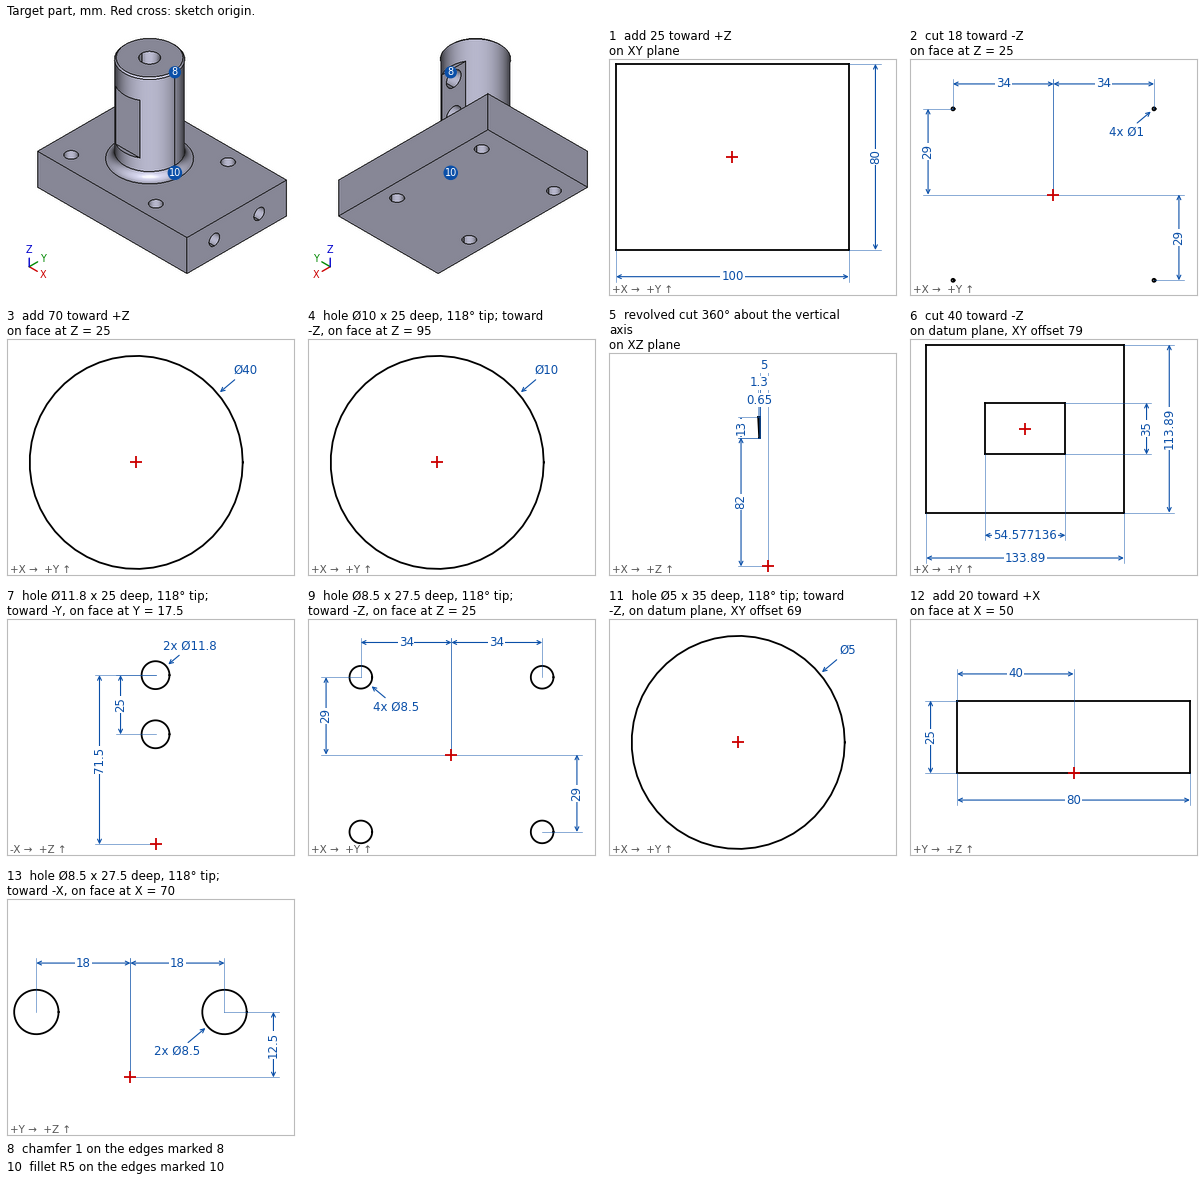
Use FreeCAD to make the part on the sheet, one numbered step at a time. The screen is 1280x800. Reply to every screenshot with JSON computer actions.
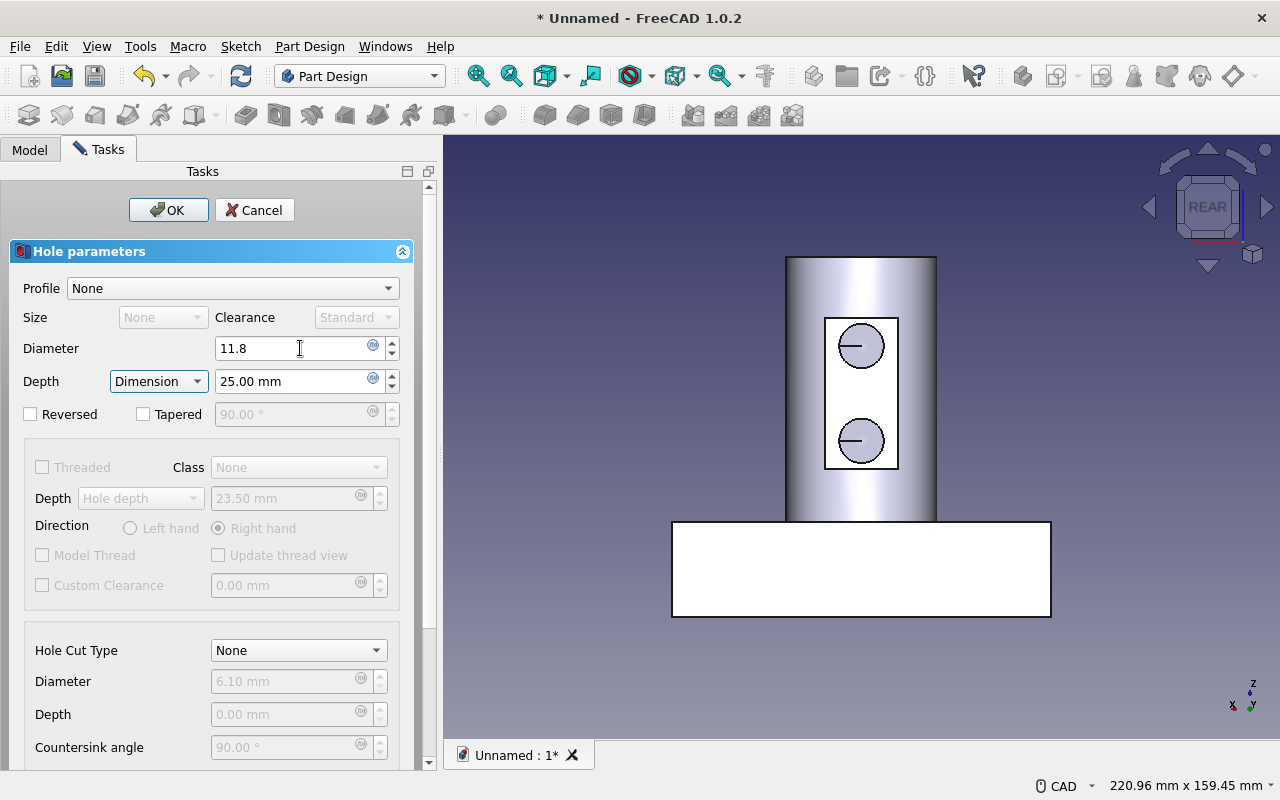
{"action": "triple_click", "coordinate": [300, 382]}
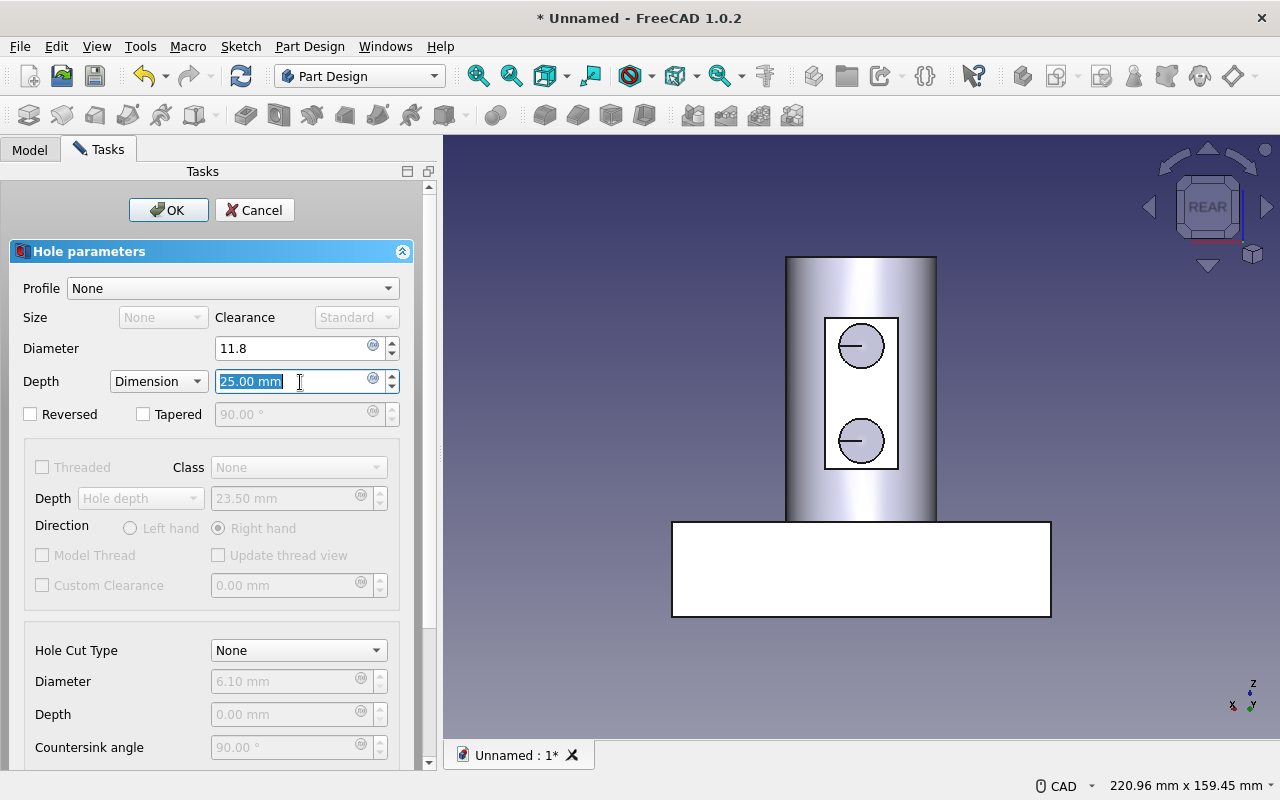
{"action": "type", "text": "25"}
{"action": "key", "text": "Tab"}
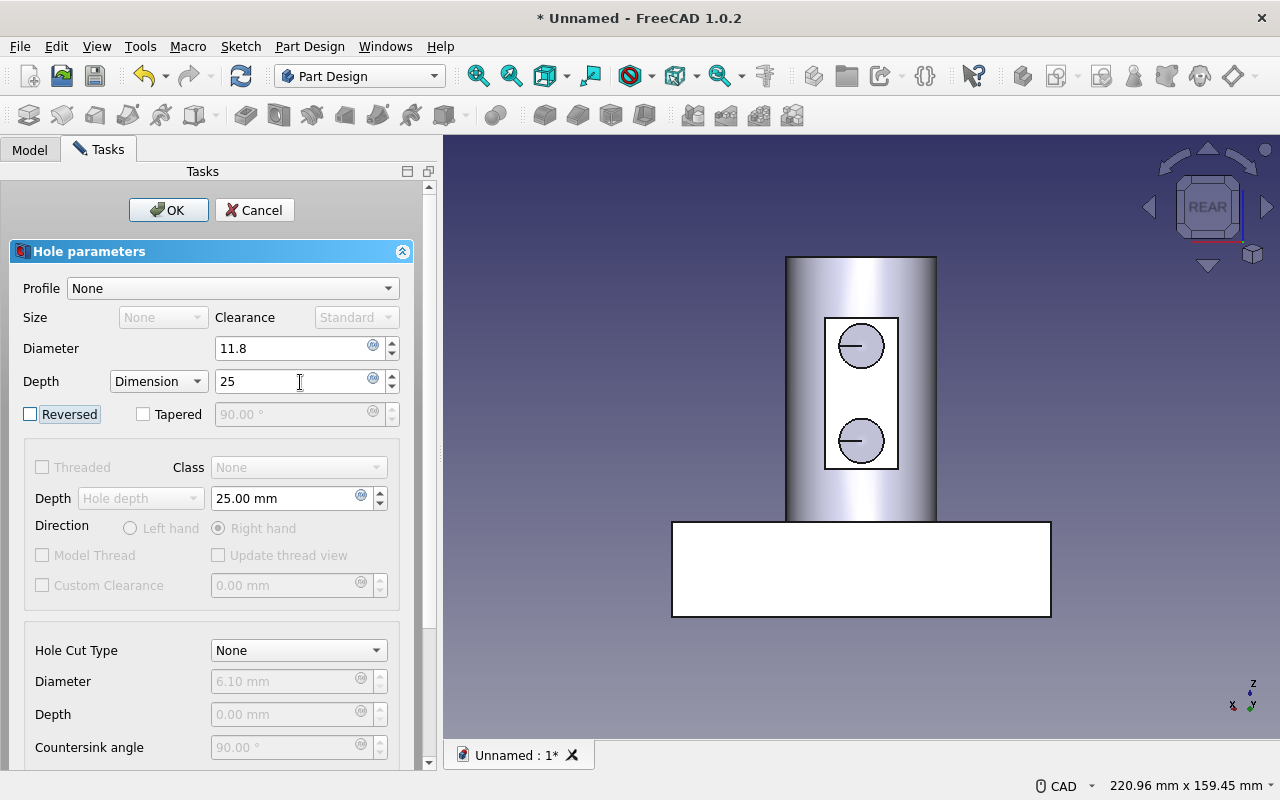
{"action": "left_click", "coordinate": [169, 210]}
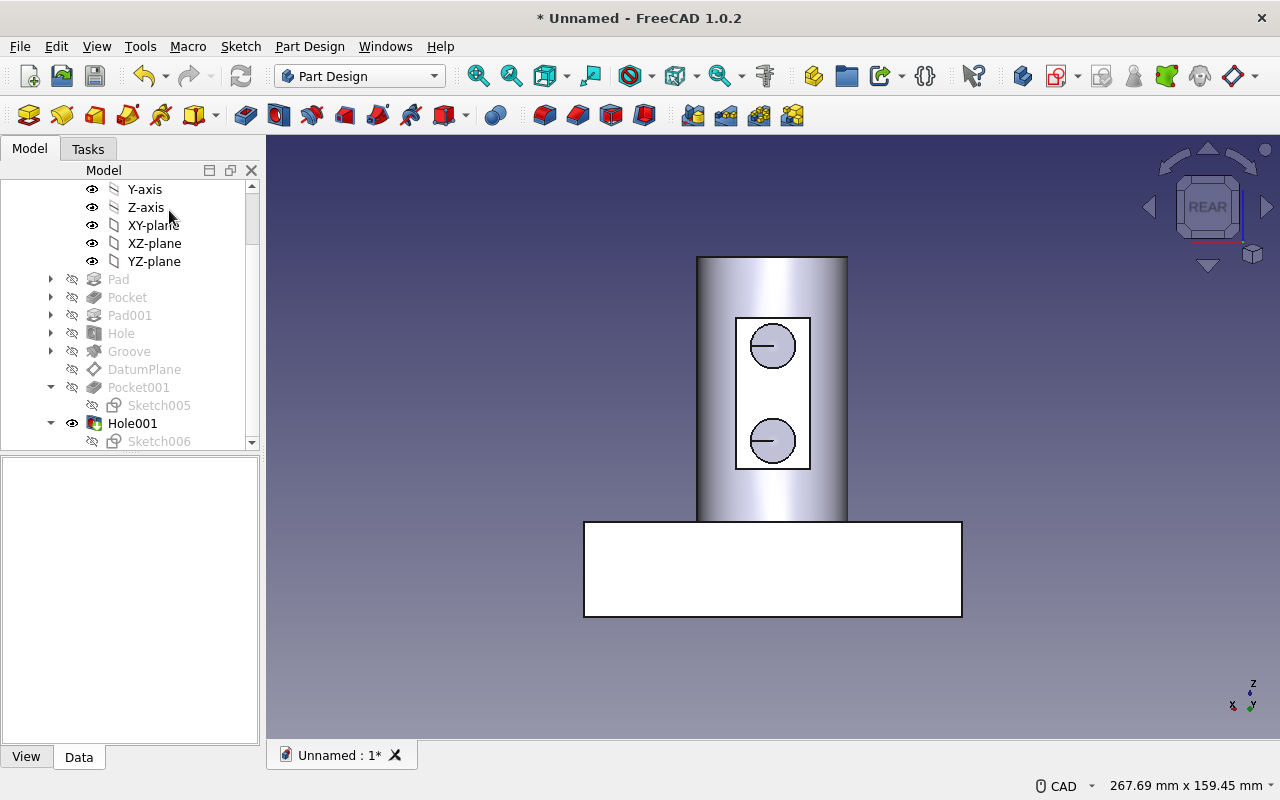
{"action": "left_click", "coordinate": [834, 256]}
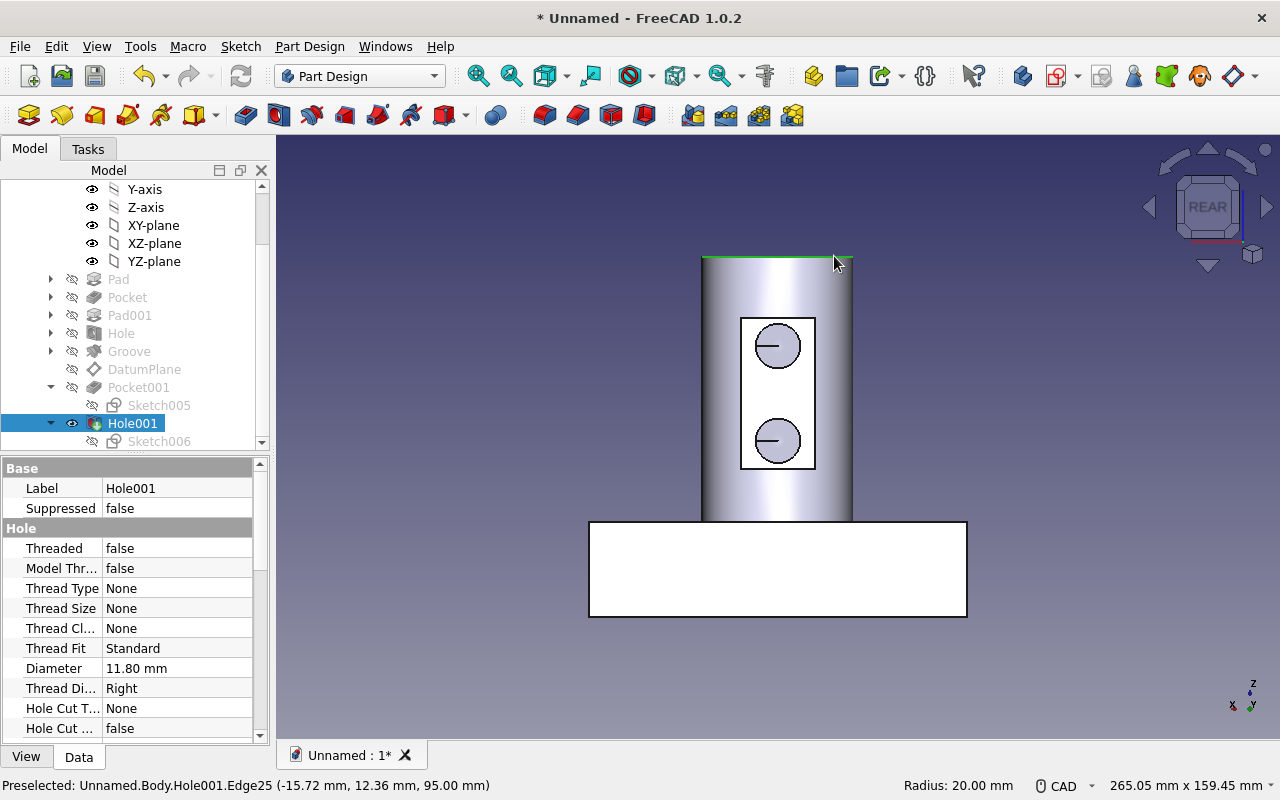
{"action": "left_click", "coordinate": [578, 116]}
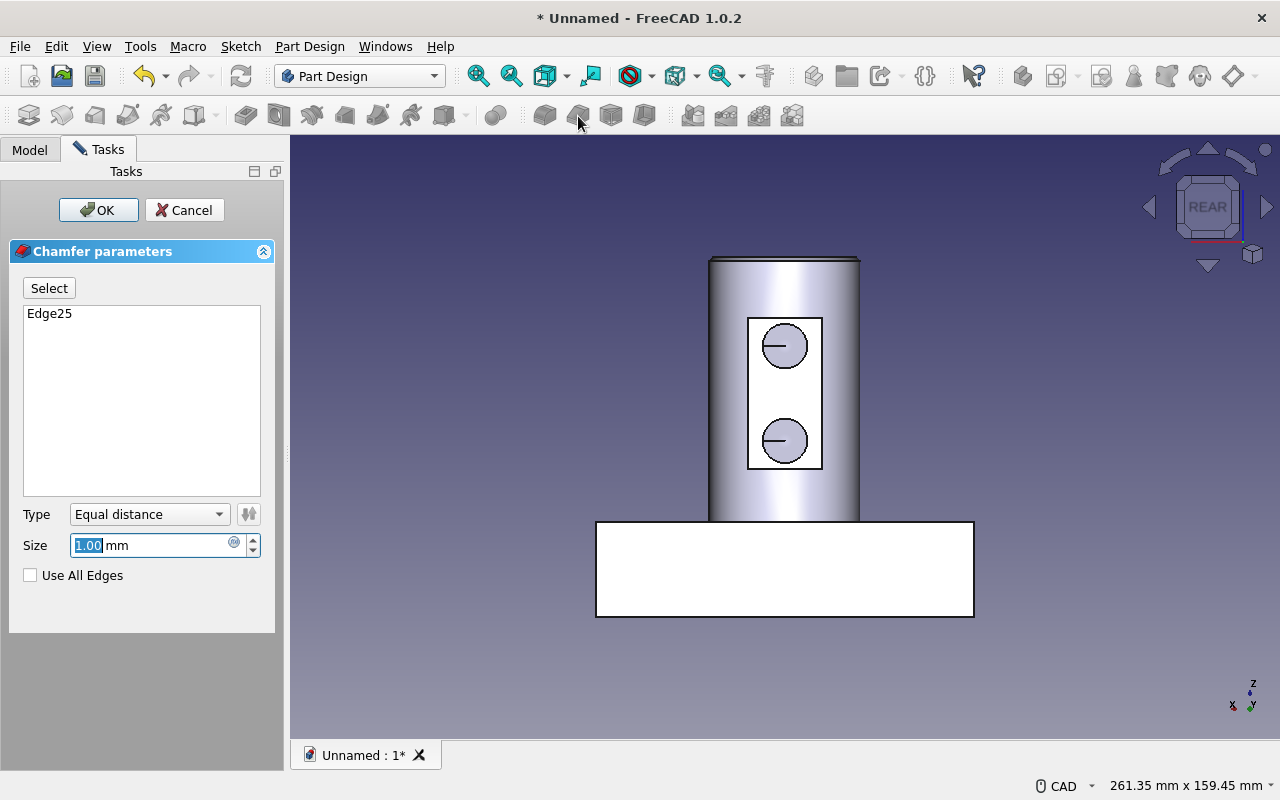
{"action": "type", "text": "1"}
{"action": "key", "text": "Tab"}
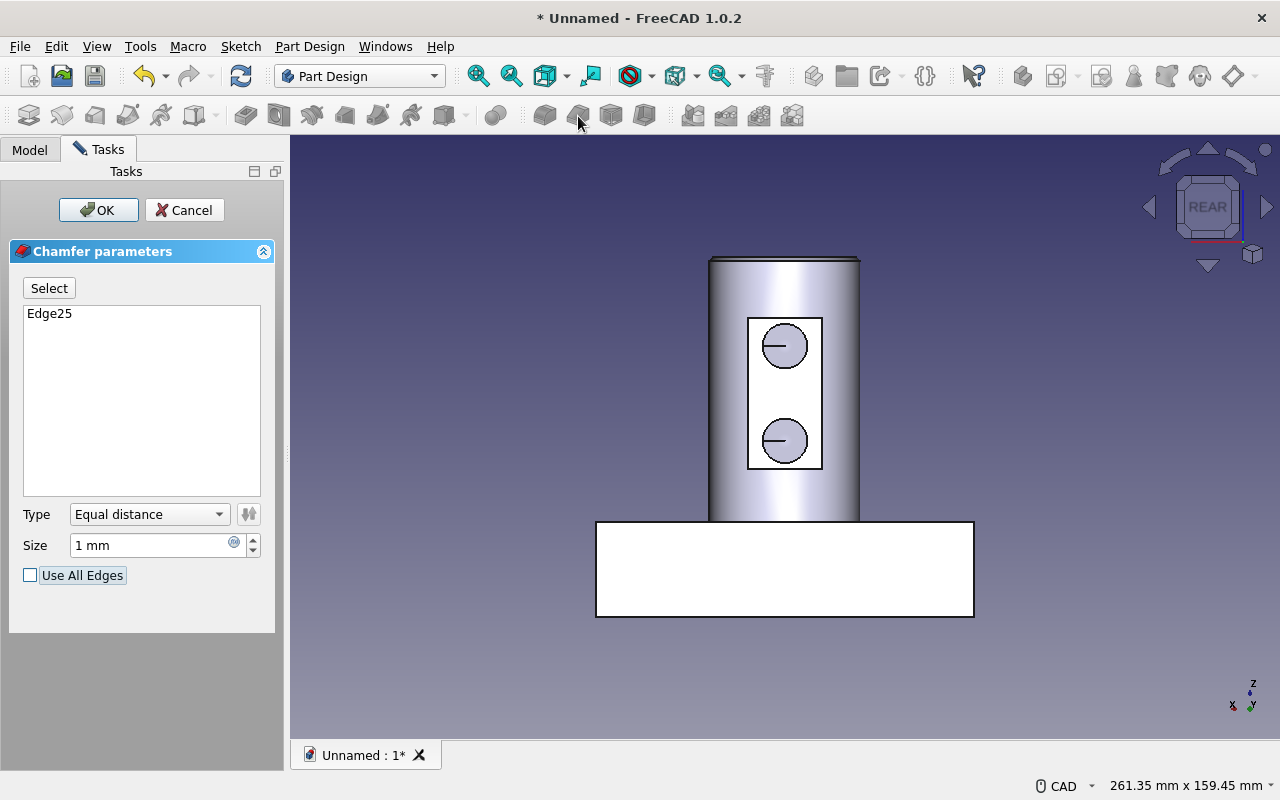
{"action": "left_click", "coordinate": [99, 210]}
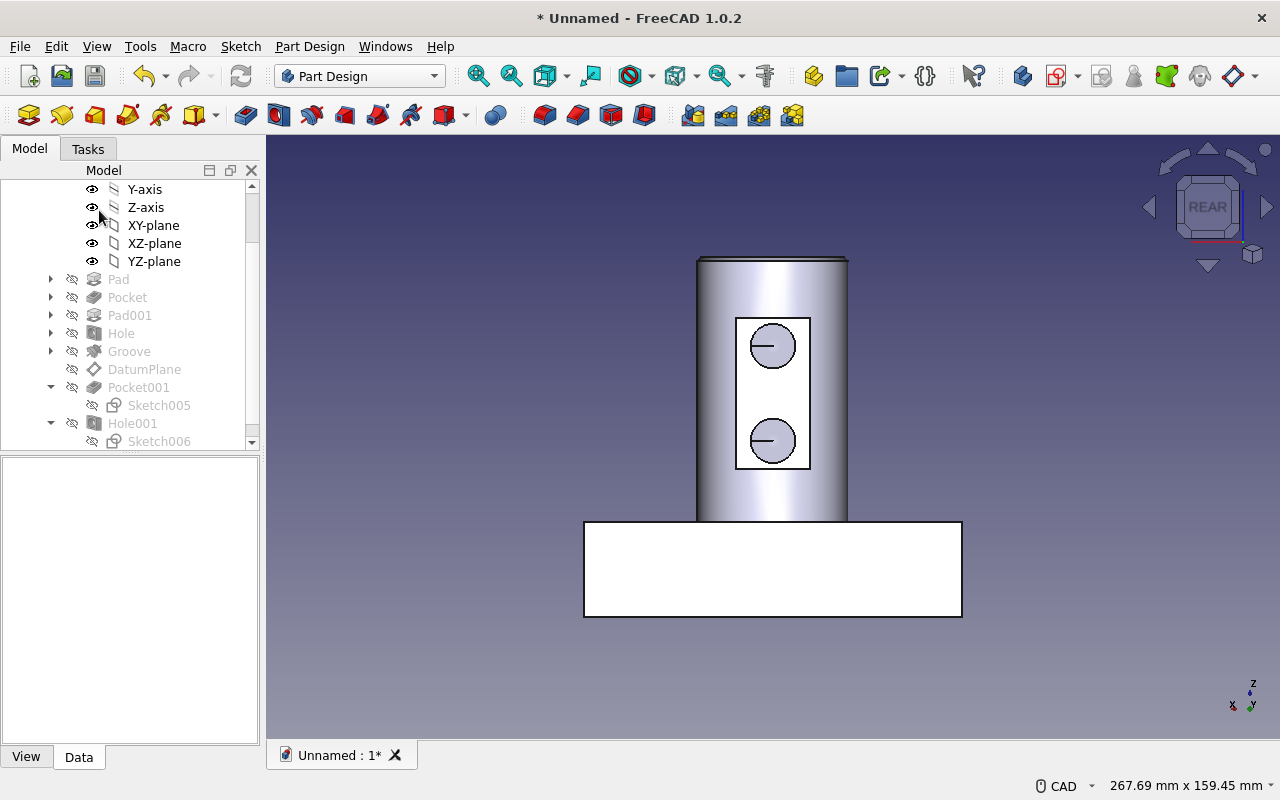
{"action": "key", "text": "0"}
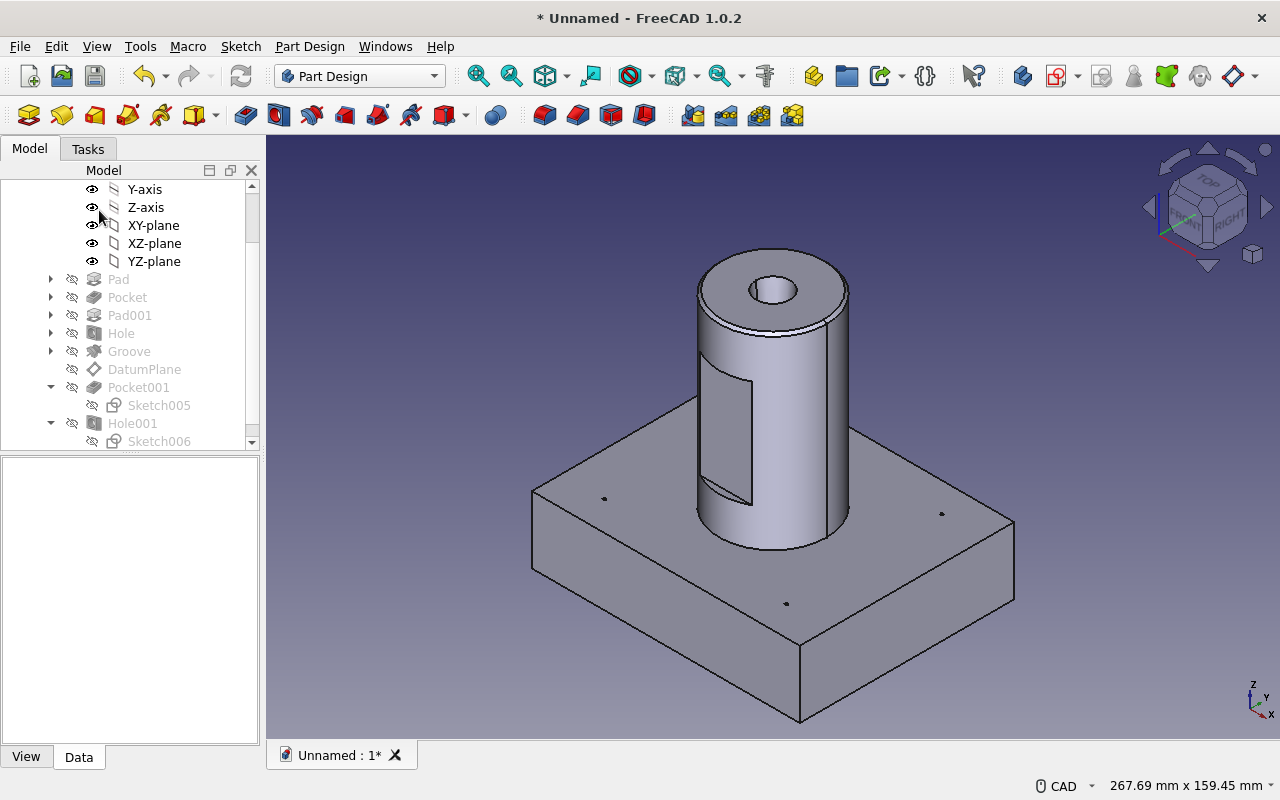
{"action": "left_click", "coordinate": [666, 479]}